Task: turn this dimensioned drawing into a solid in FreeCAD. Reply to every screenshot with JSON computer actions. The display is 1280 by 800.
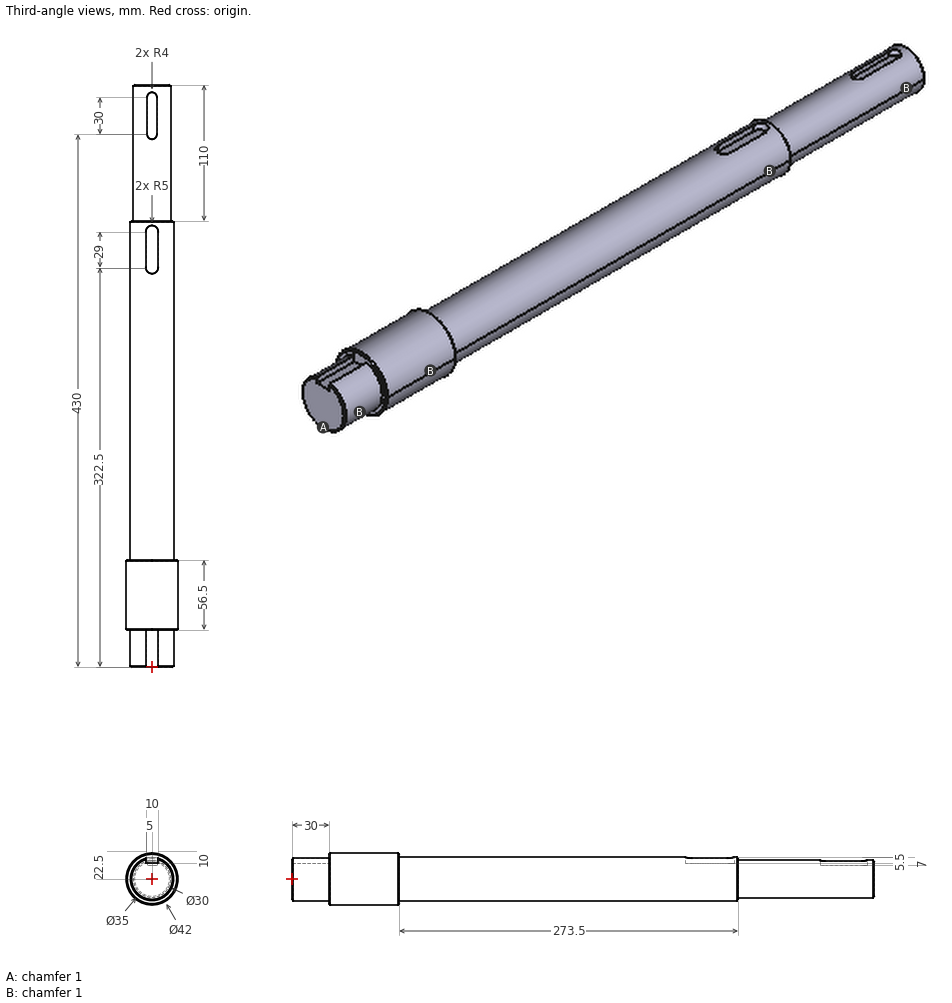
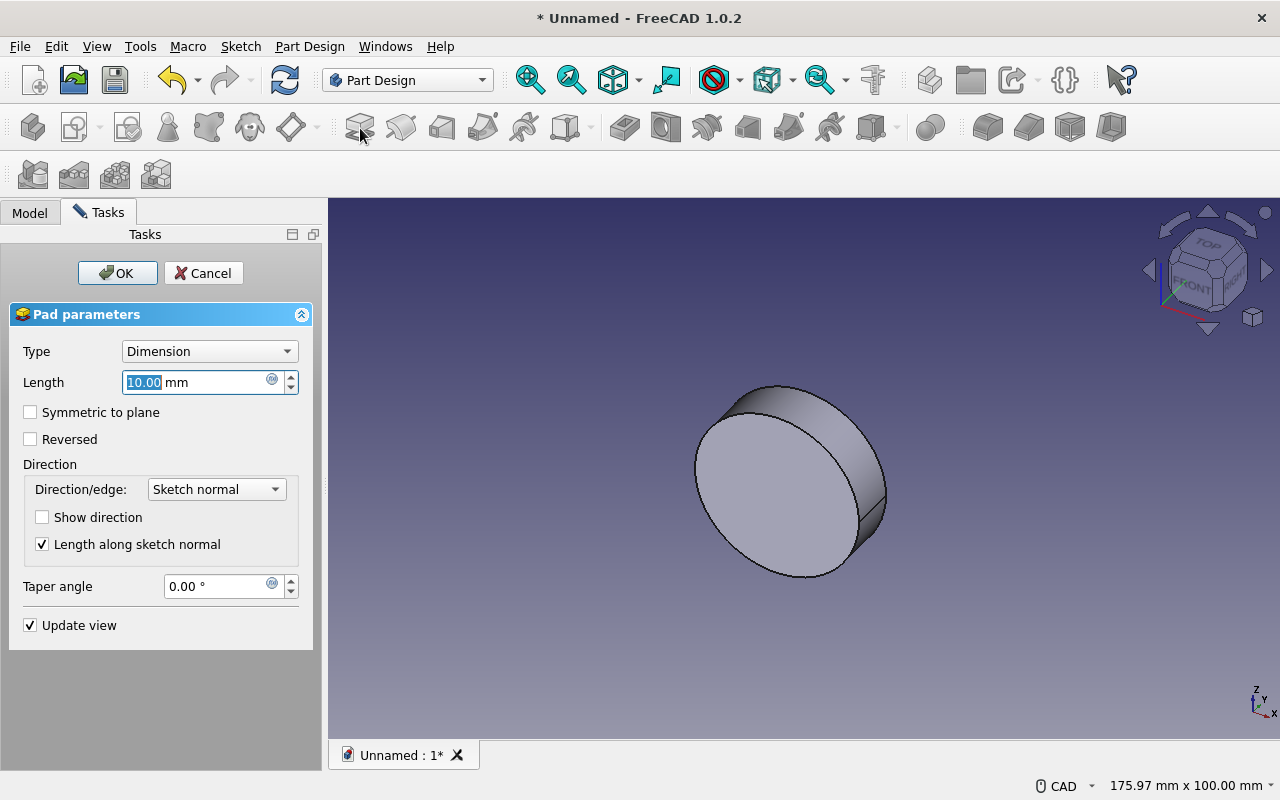
{"action": "type", "text": "30"}
{"action": "key", "text": "Tab"}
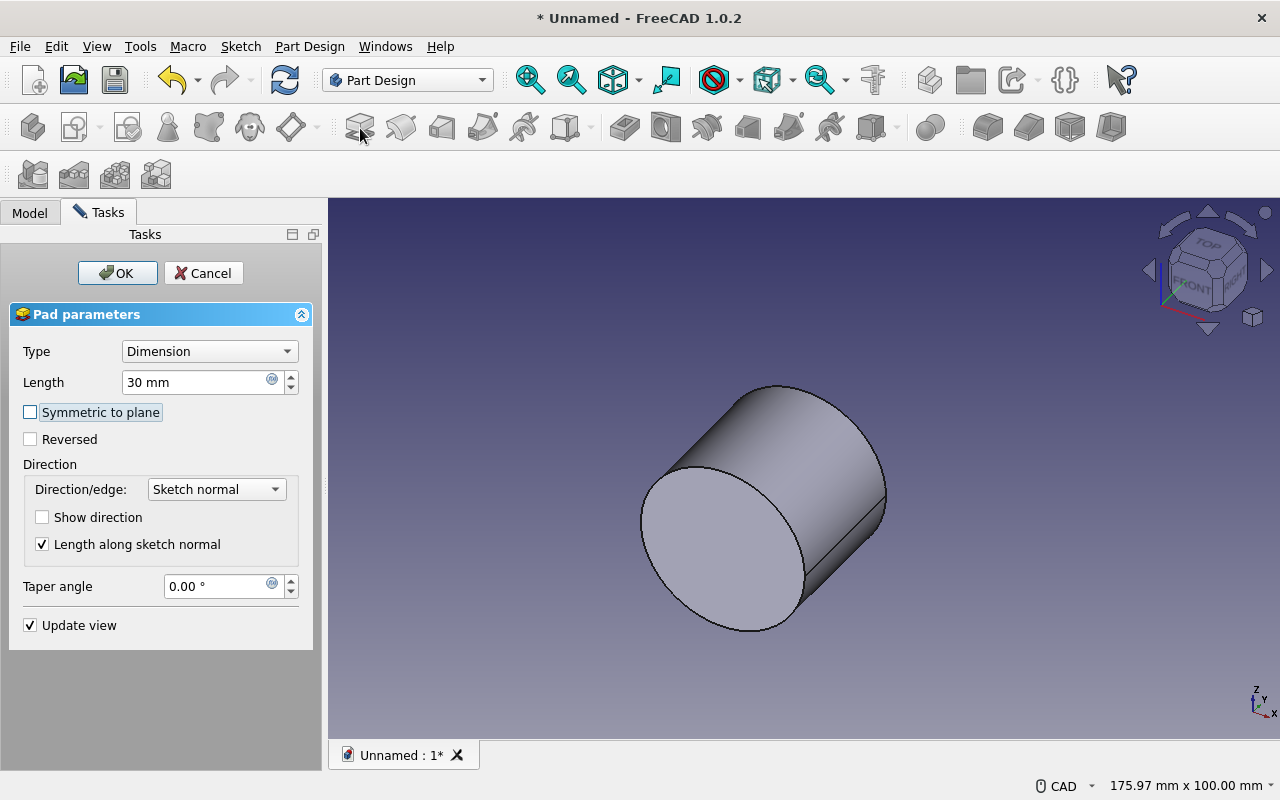
{"action": "left_click", "coordinate": [31, 439]}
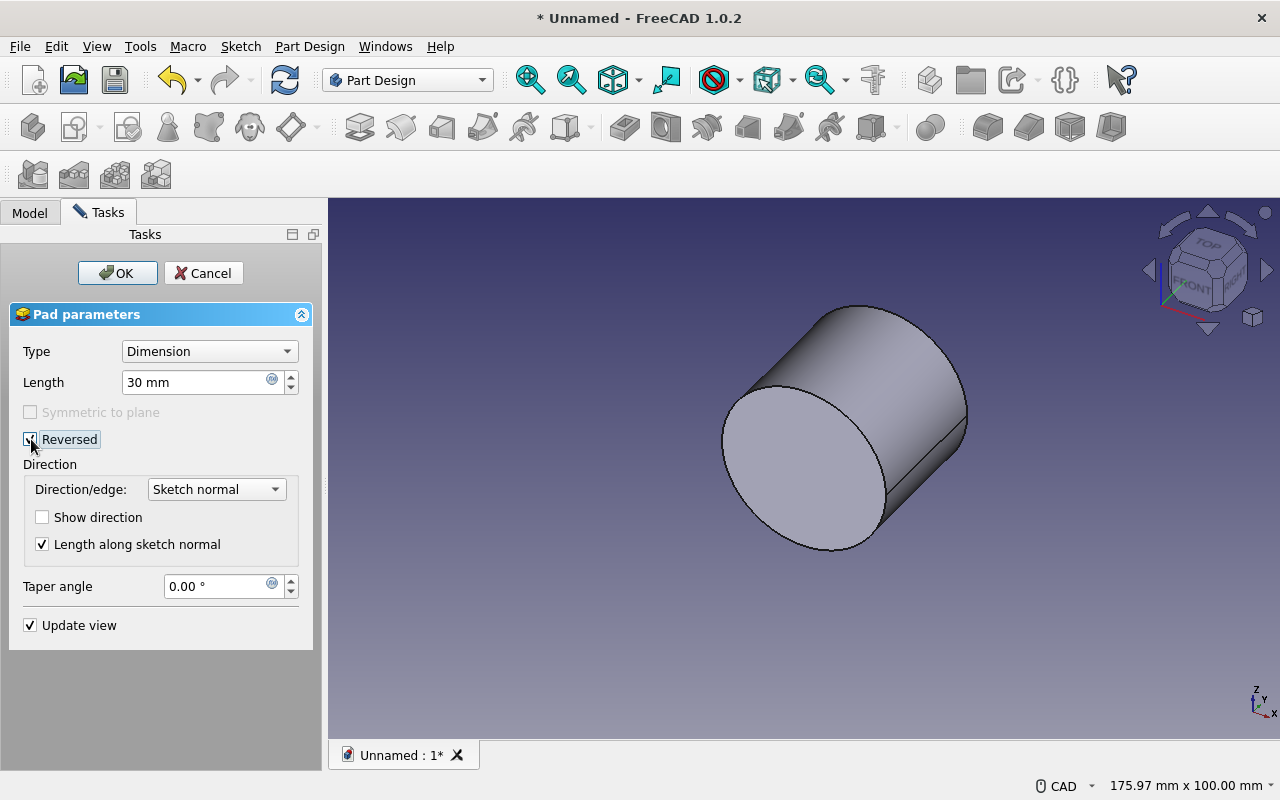
{"action": "left_click", "coordinate": [118, 273]}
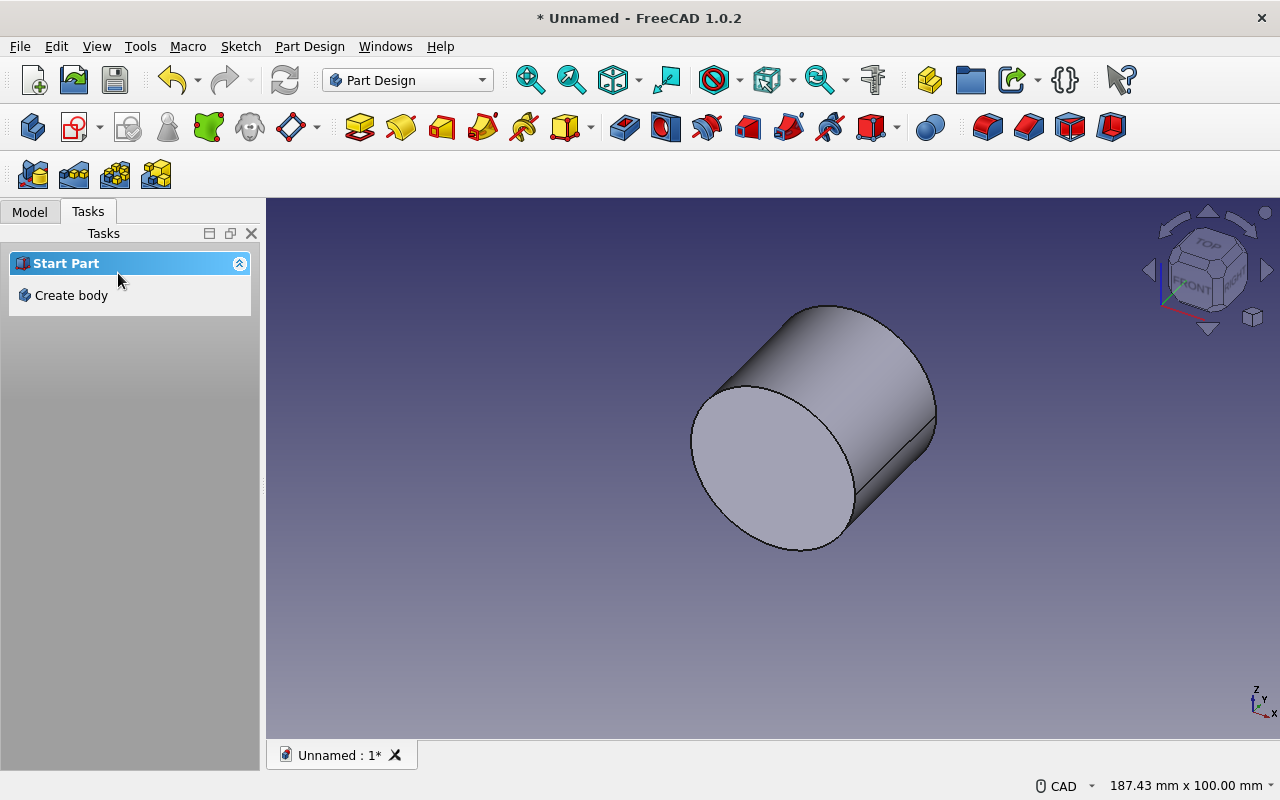
{"action": "key", "text": "4"}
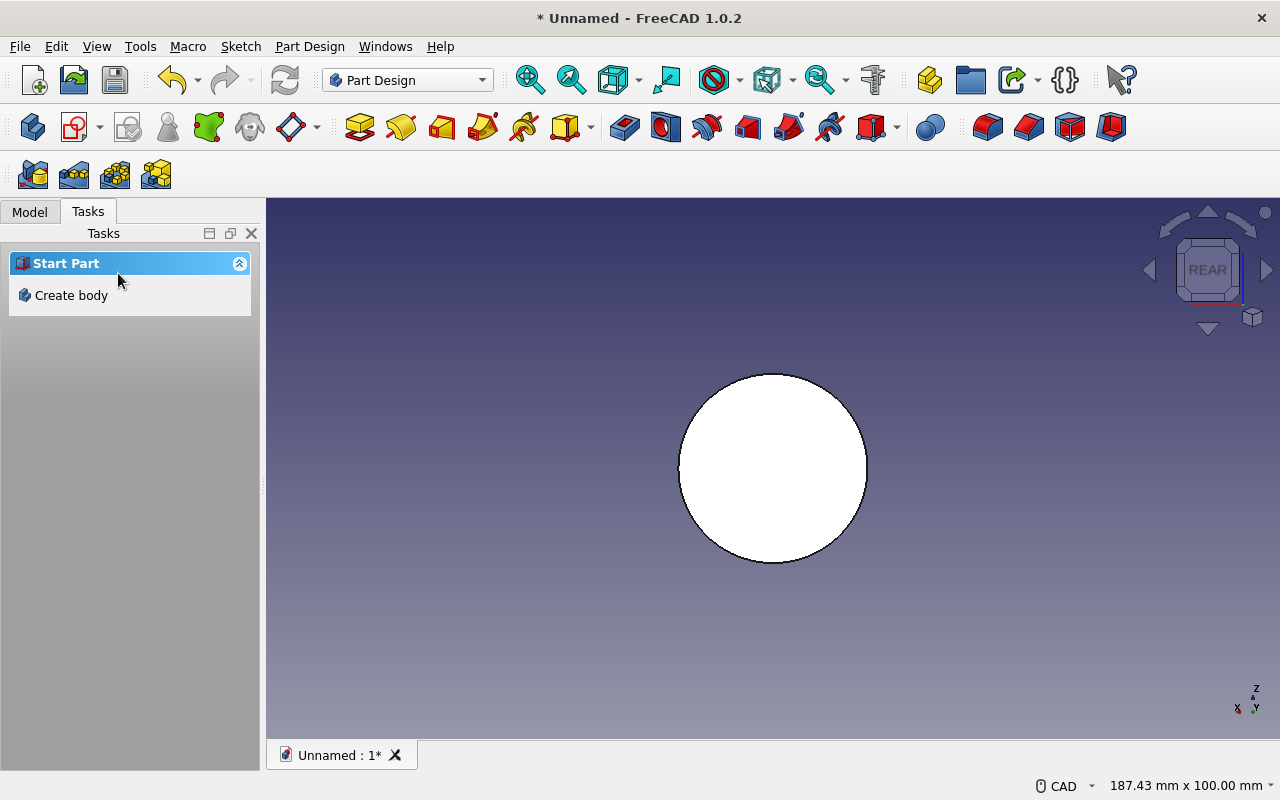
{"action": "left_click", "coordinate": [531, 80]}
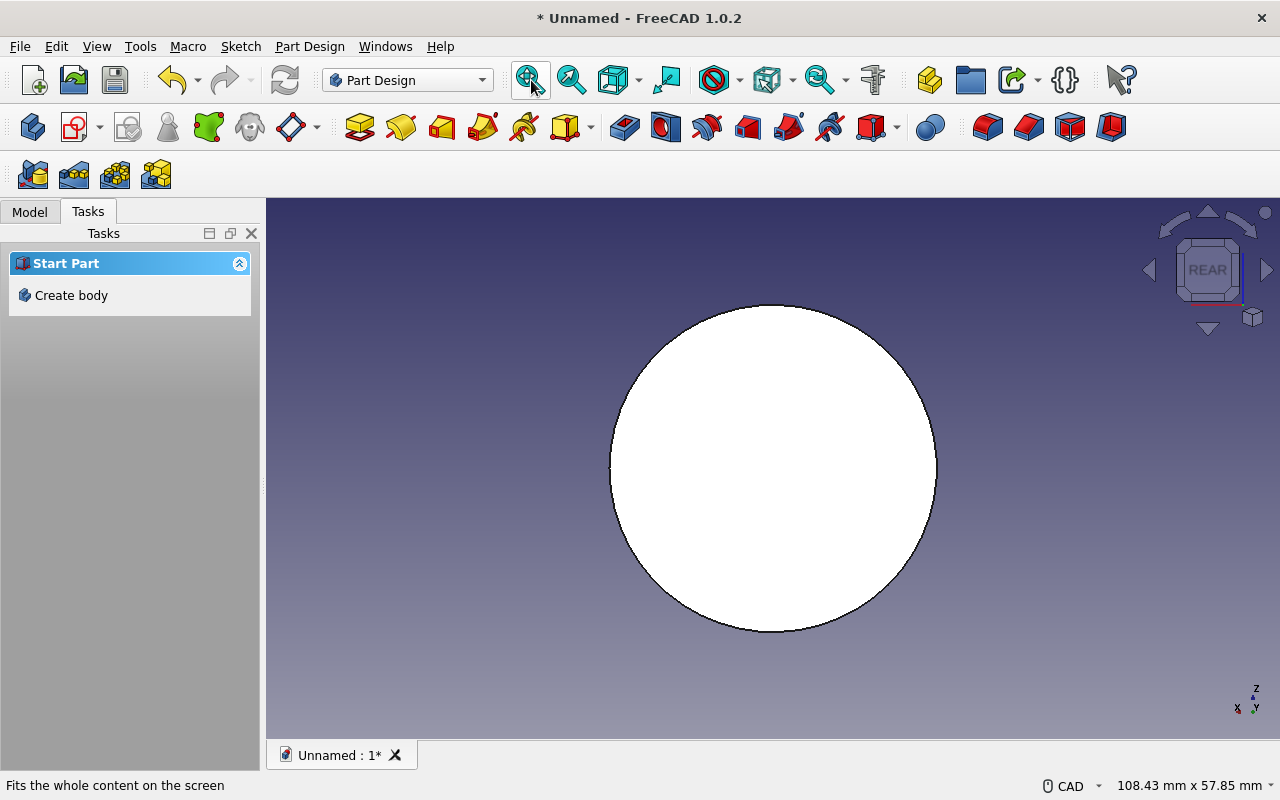
{"action": "left_click", "coordinate": [773, 468]}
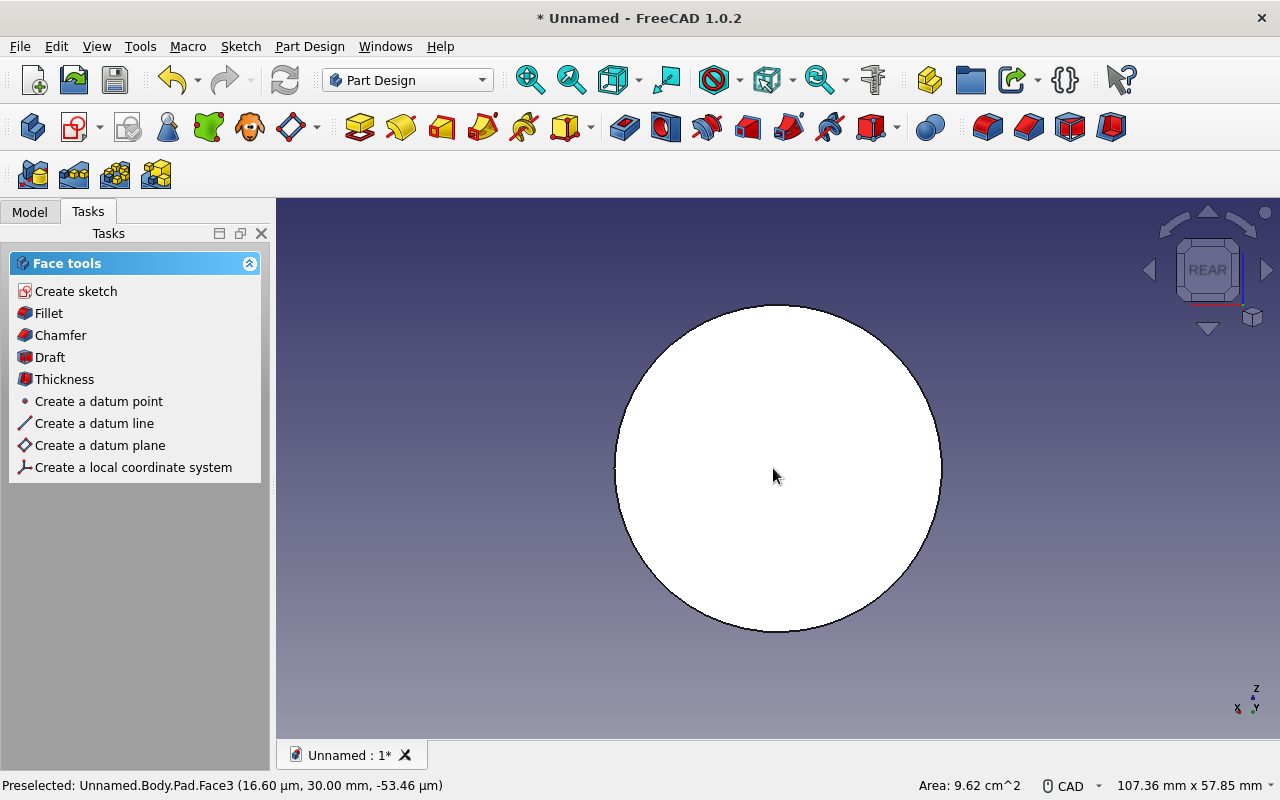
{"action": "left_click", "coordinate": [74, 128]}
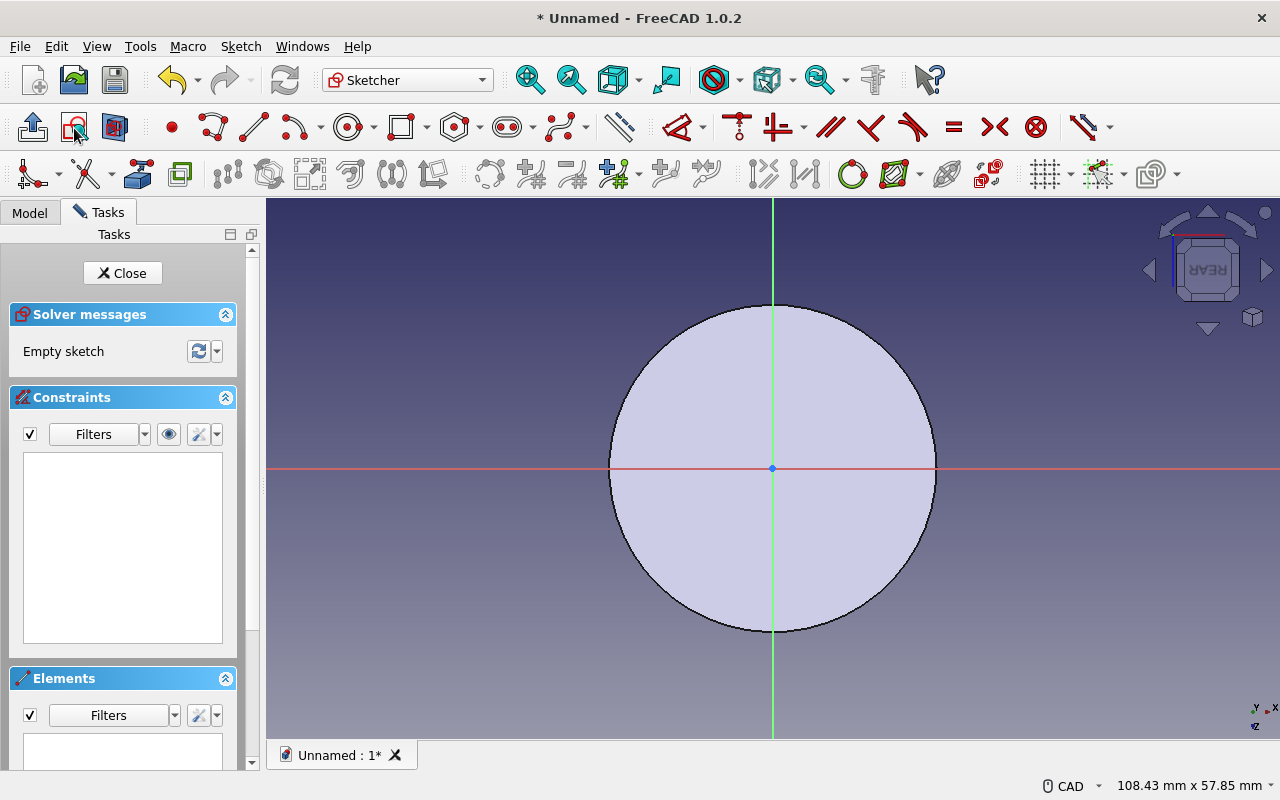
{"action": "key", "text": "g c"}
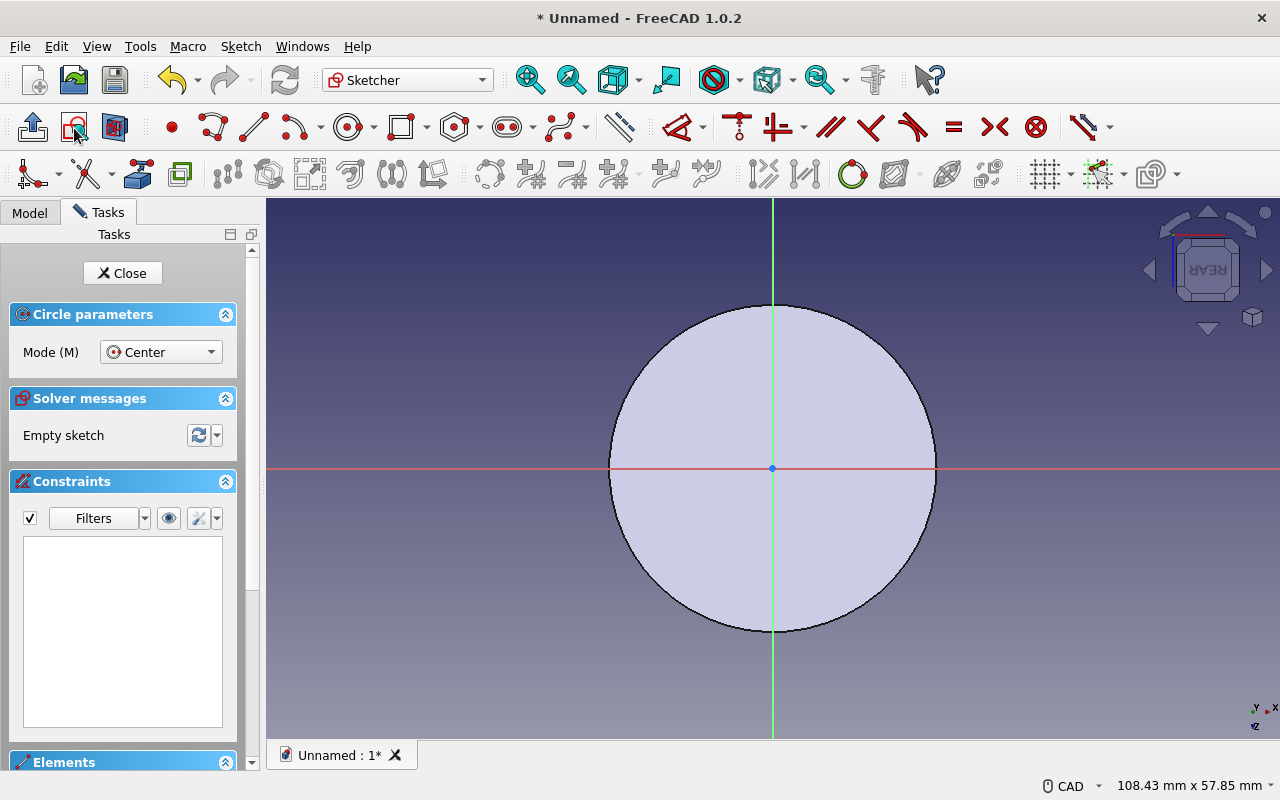
{"action": "left_click", "coordinate": [773, 468]}
{"action": "mouse_move", "coordinate": [912, 330]}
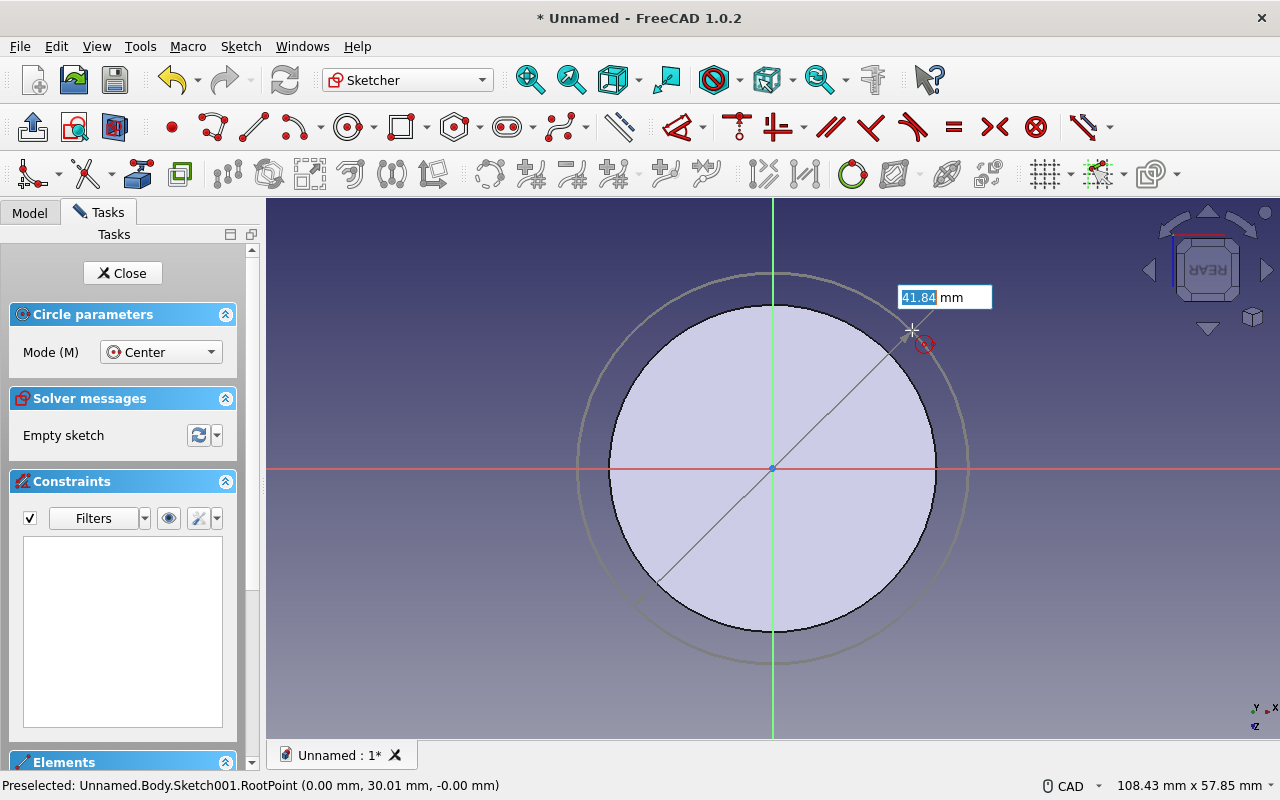
{"action": "type", "text": "42"}
{"action": "key", "text": "Return"}
{"action": "key", "text": "Escape"}